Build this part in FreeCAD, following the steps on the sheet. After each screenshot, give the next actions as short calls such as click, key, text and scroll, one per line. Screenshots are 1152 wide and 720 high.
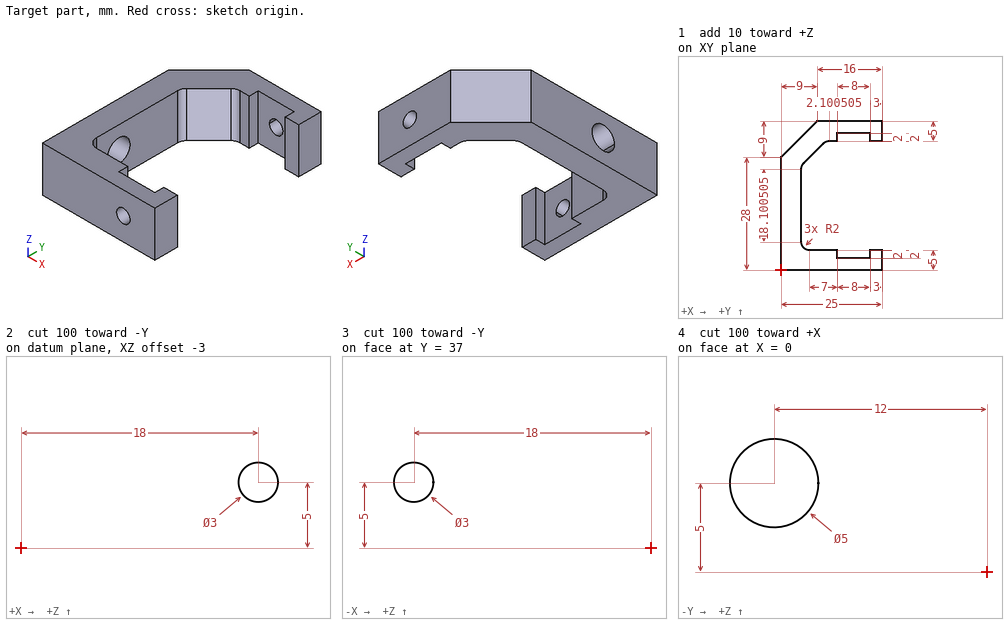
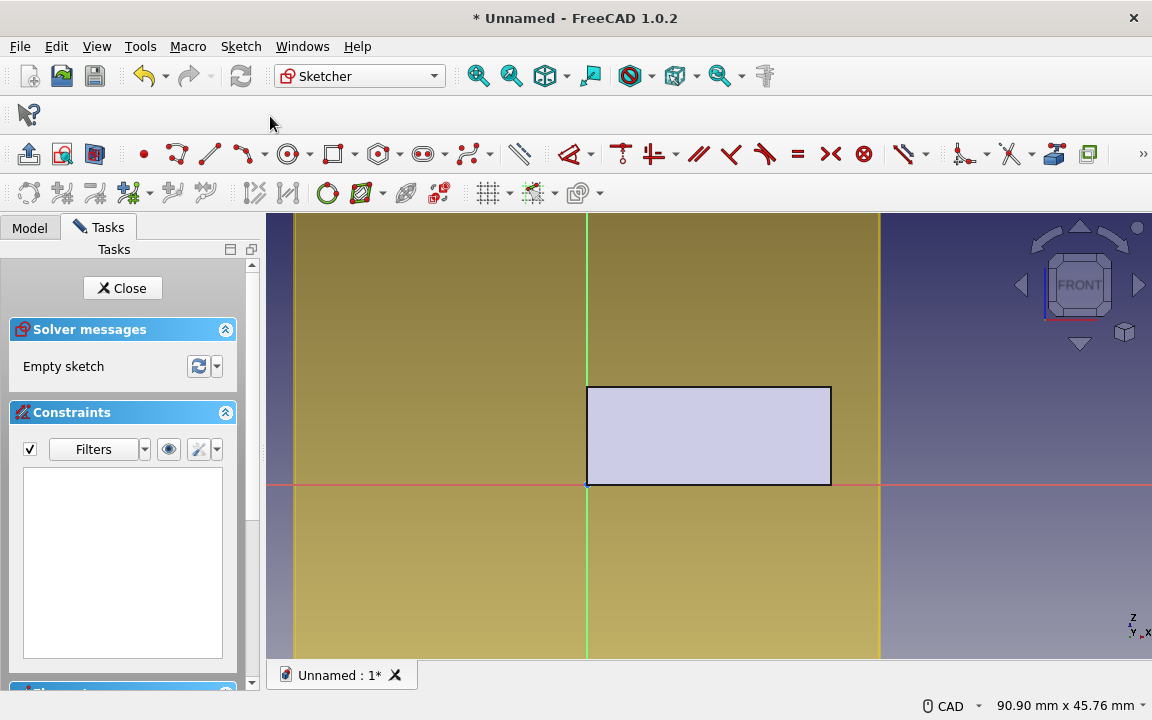
key(q)
key(s)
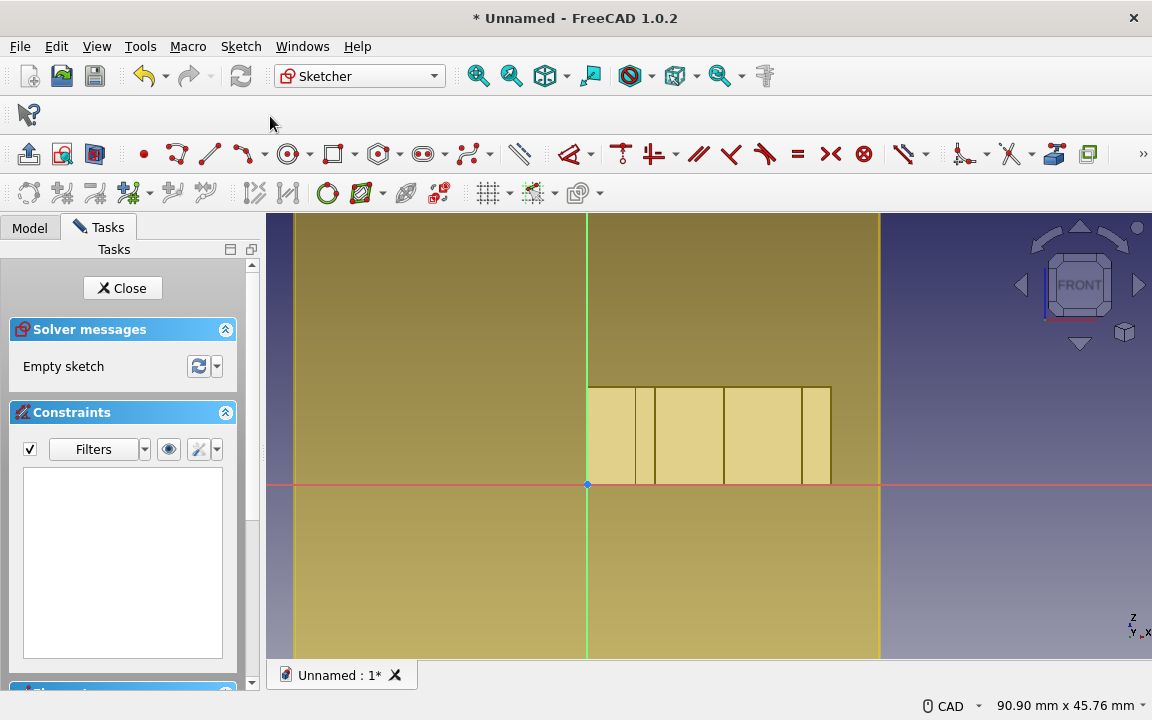
scroll(778, 436, up, 11)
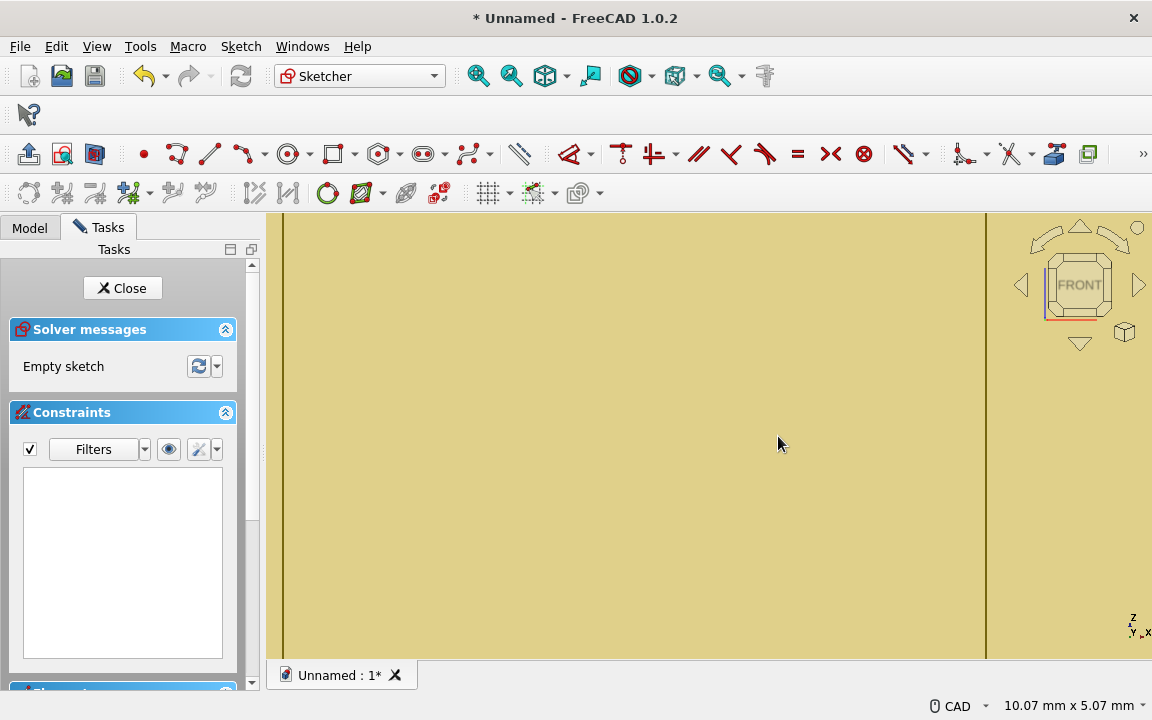
key(g)
key(c)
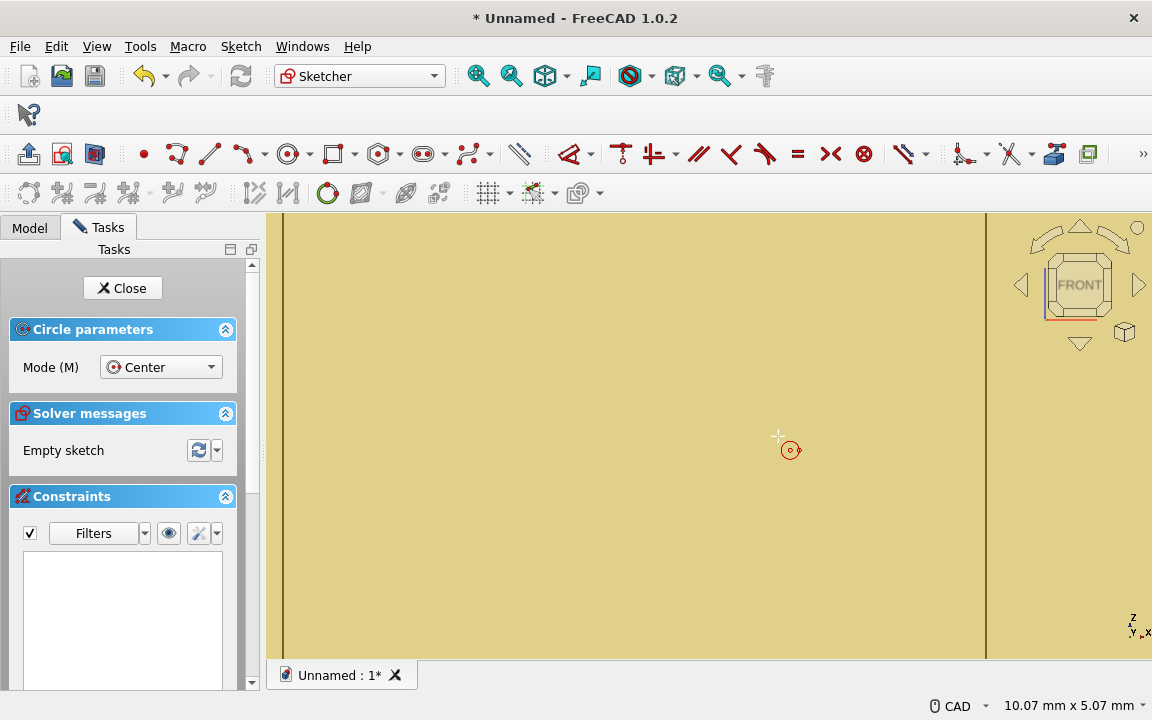
click(634, 432)
click(728, 339)
key(Escape)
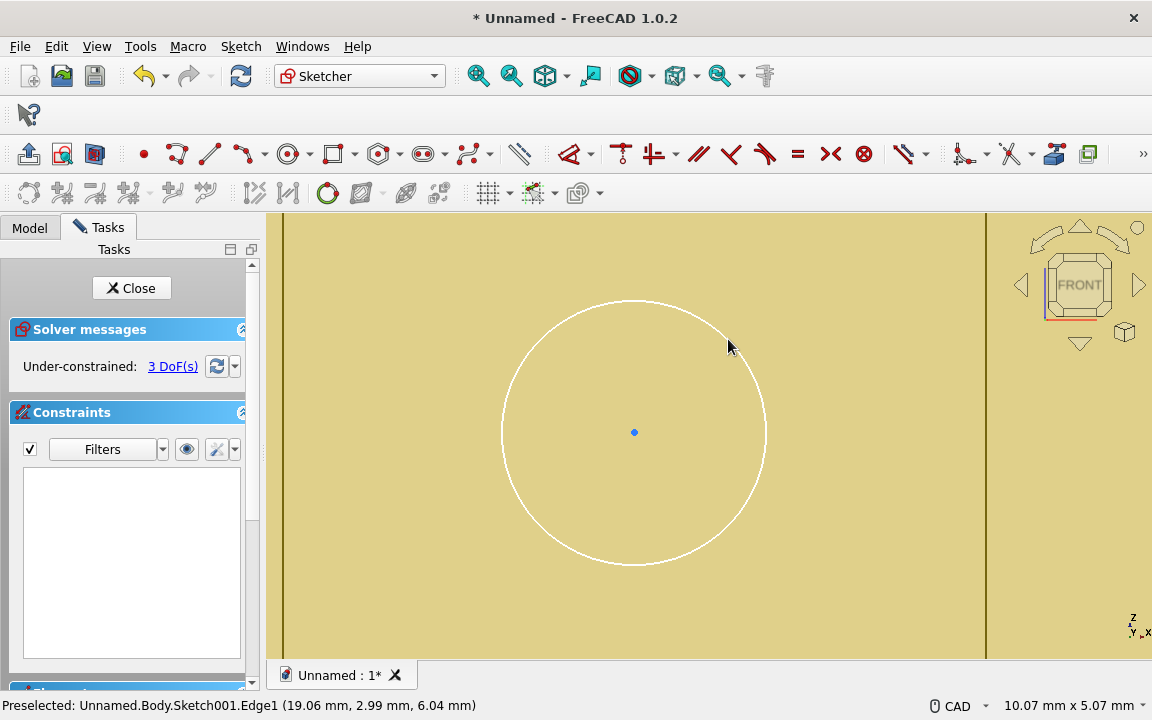
click(568, 154)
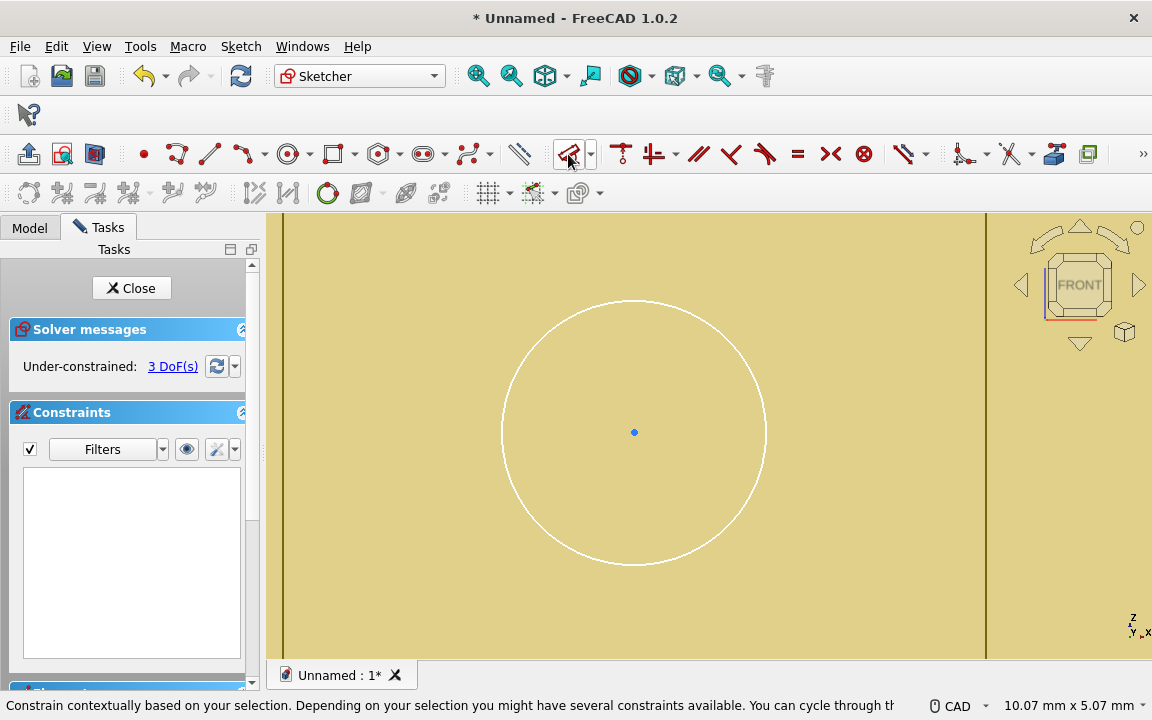
click(727, 339)
click(750, 316)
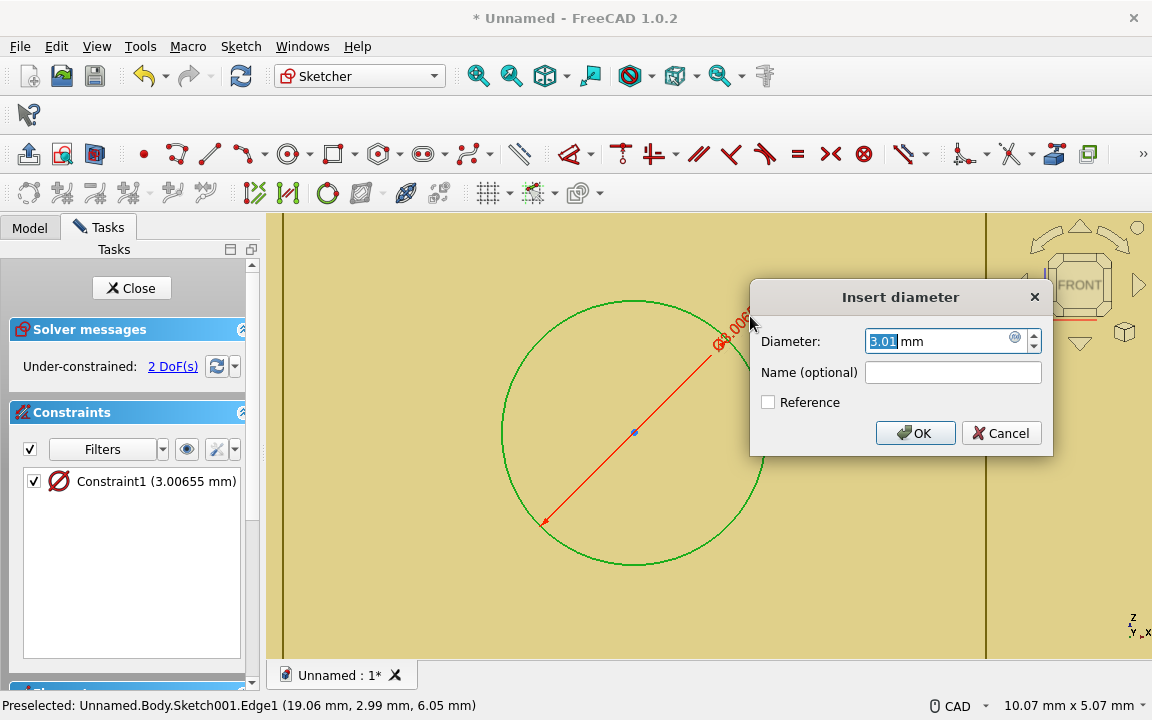
text(3)
key(Return)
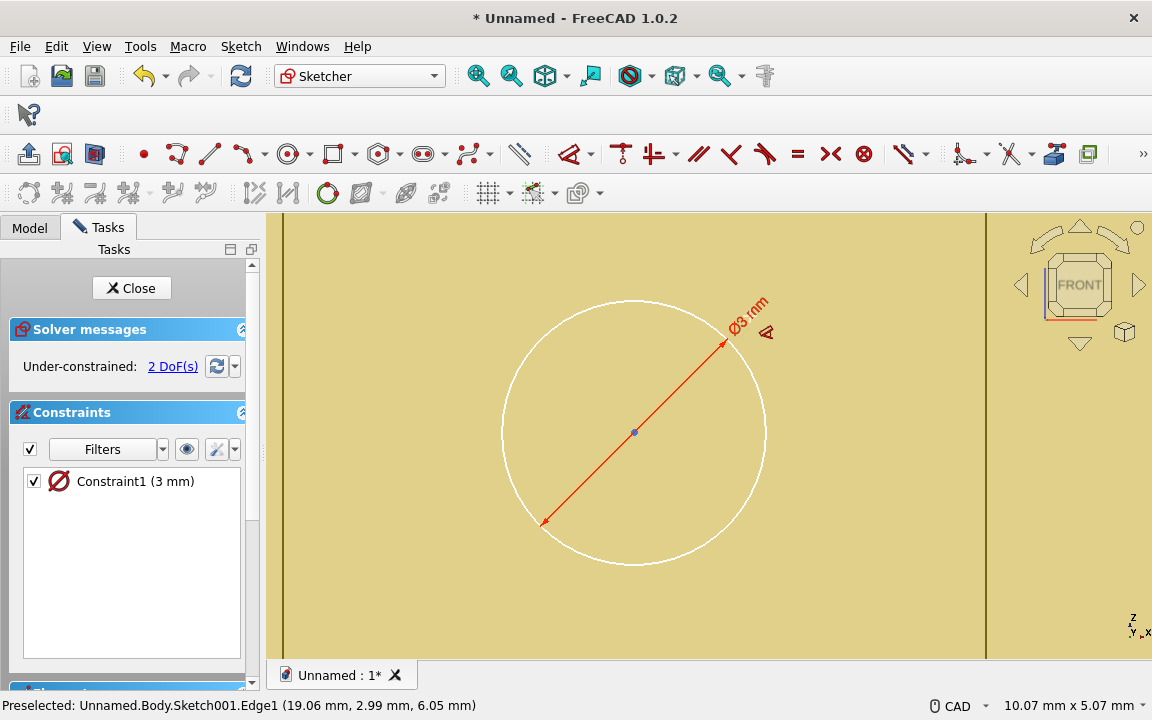
click(634, 433)
click(668, 532)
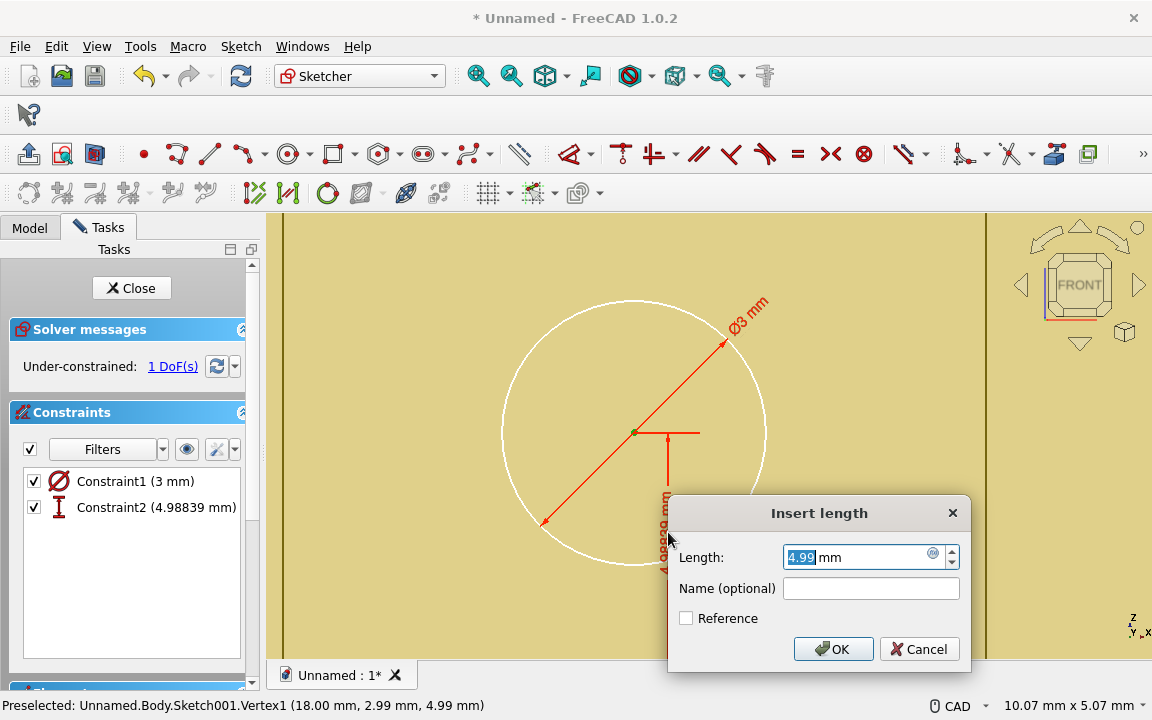
text(5)
key(Return)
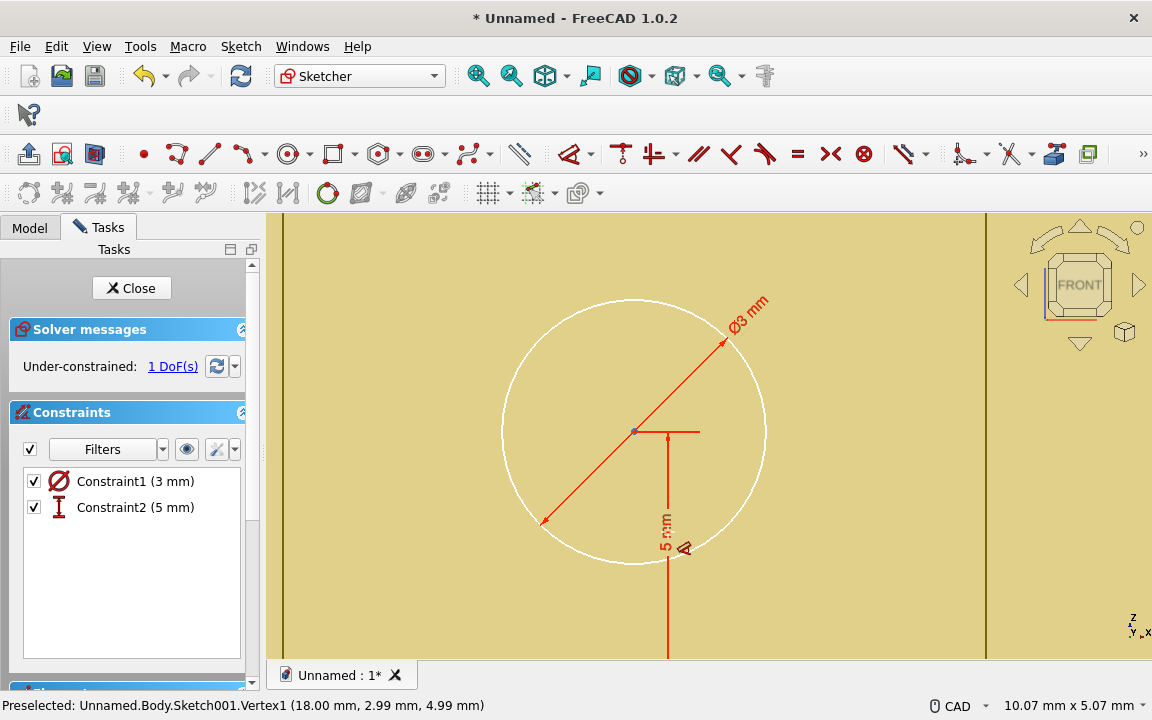
click(634, 432)
click(464, 398)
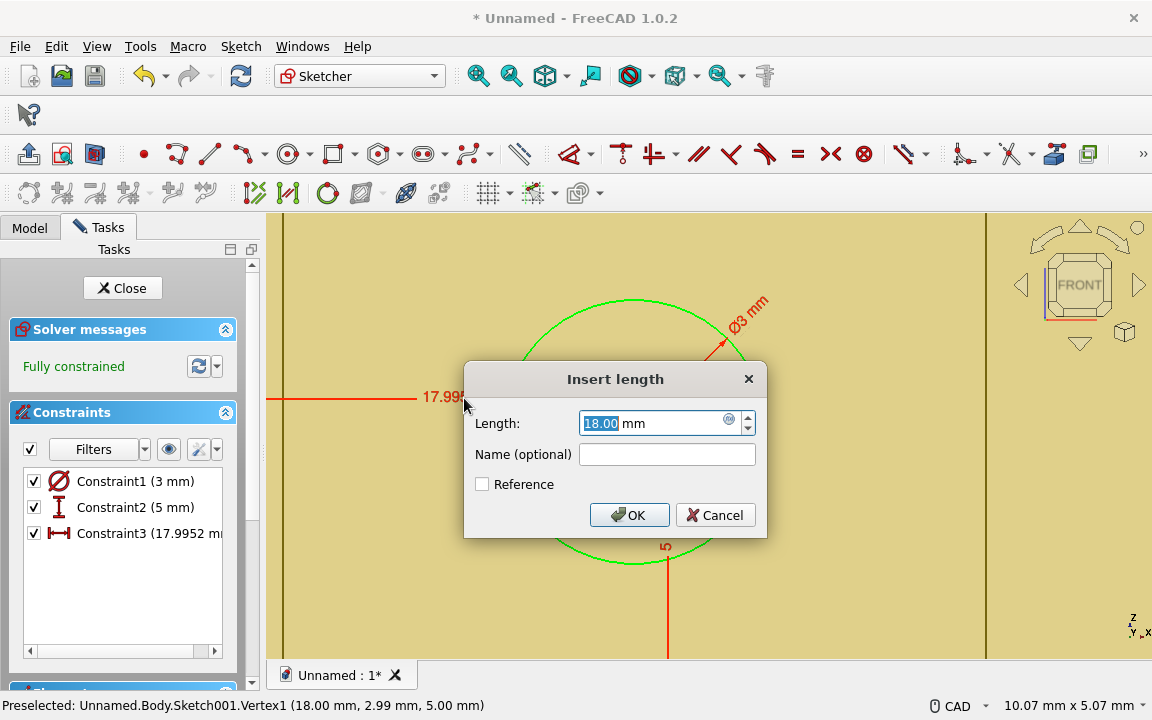
text(18)
key(Return)
key(Escape)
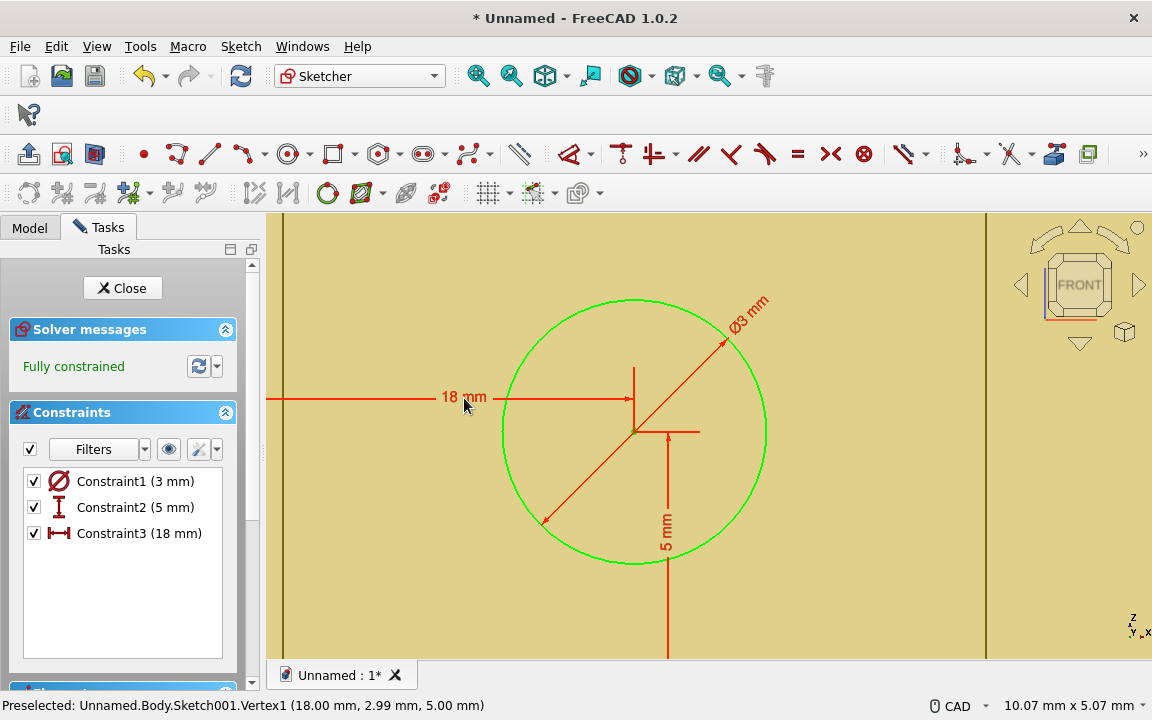
click(123, 288)